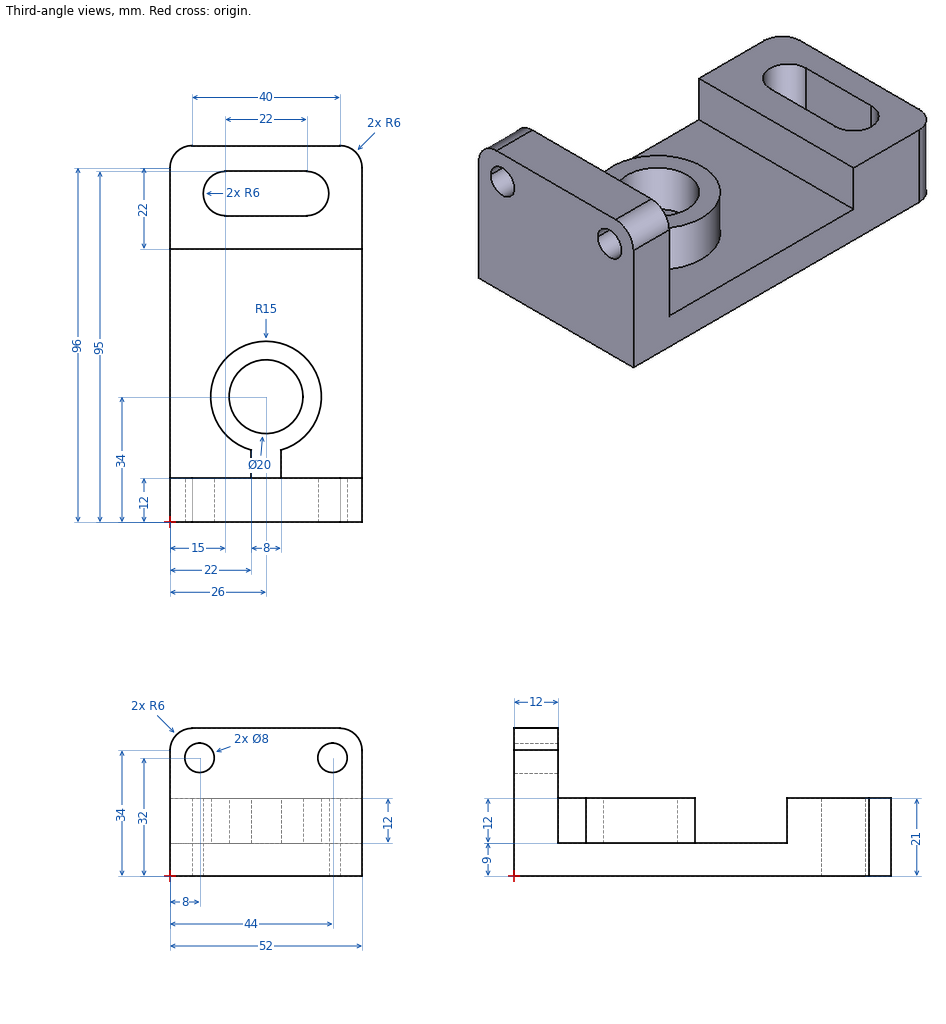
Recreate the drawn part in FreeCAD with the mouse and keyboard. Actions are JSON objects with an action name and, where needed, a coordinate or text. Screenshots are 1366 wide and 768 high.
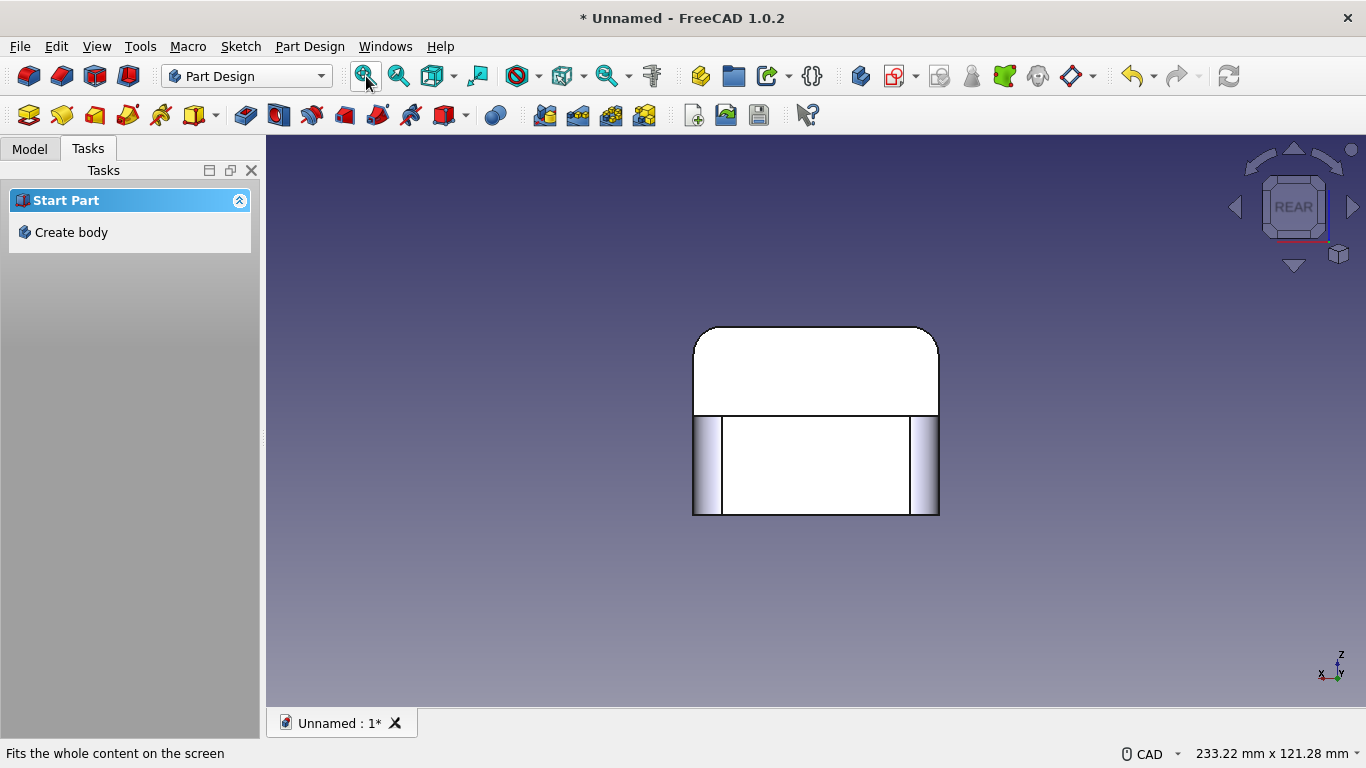
{"action": "left_click", "coordinate": [366, 76]}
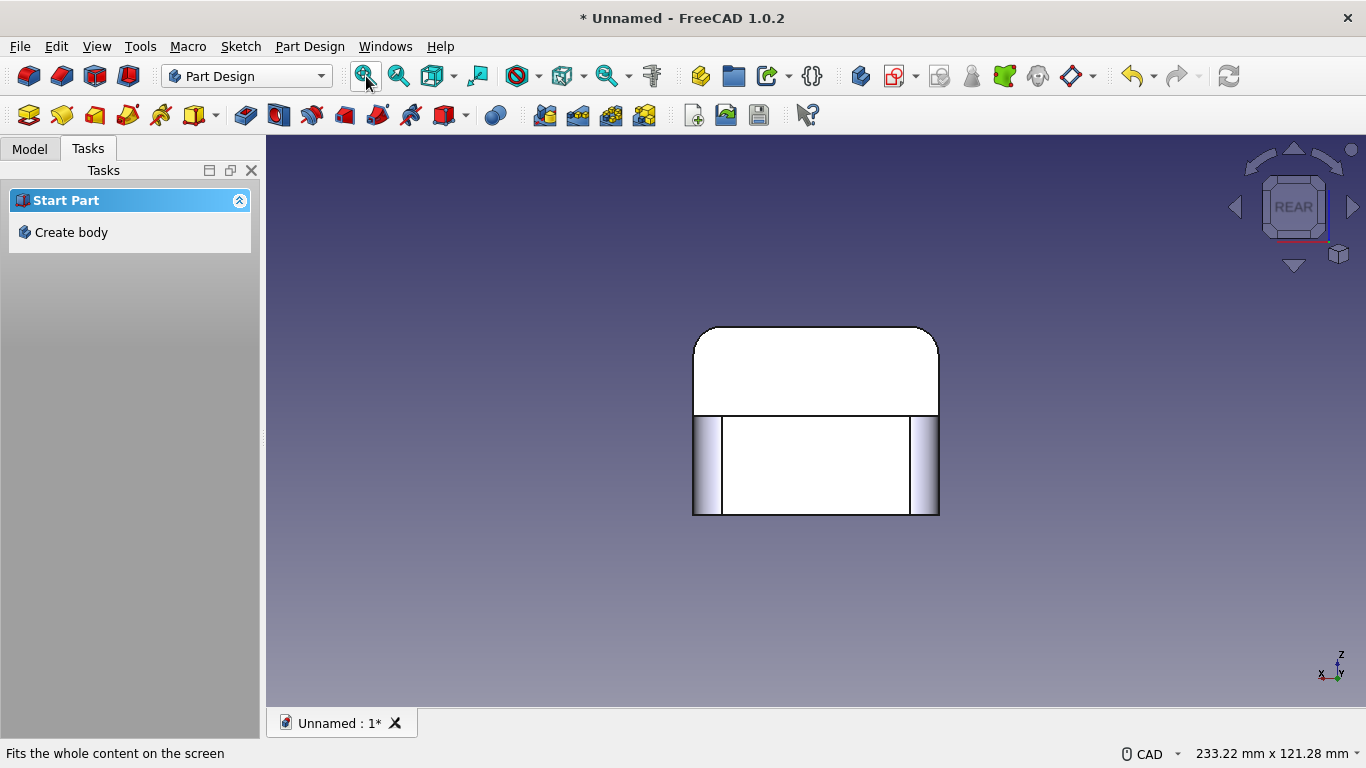
{"action": "left_click", "coordinate": [781, 399]}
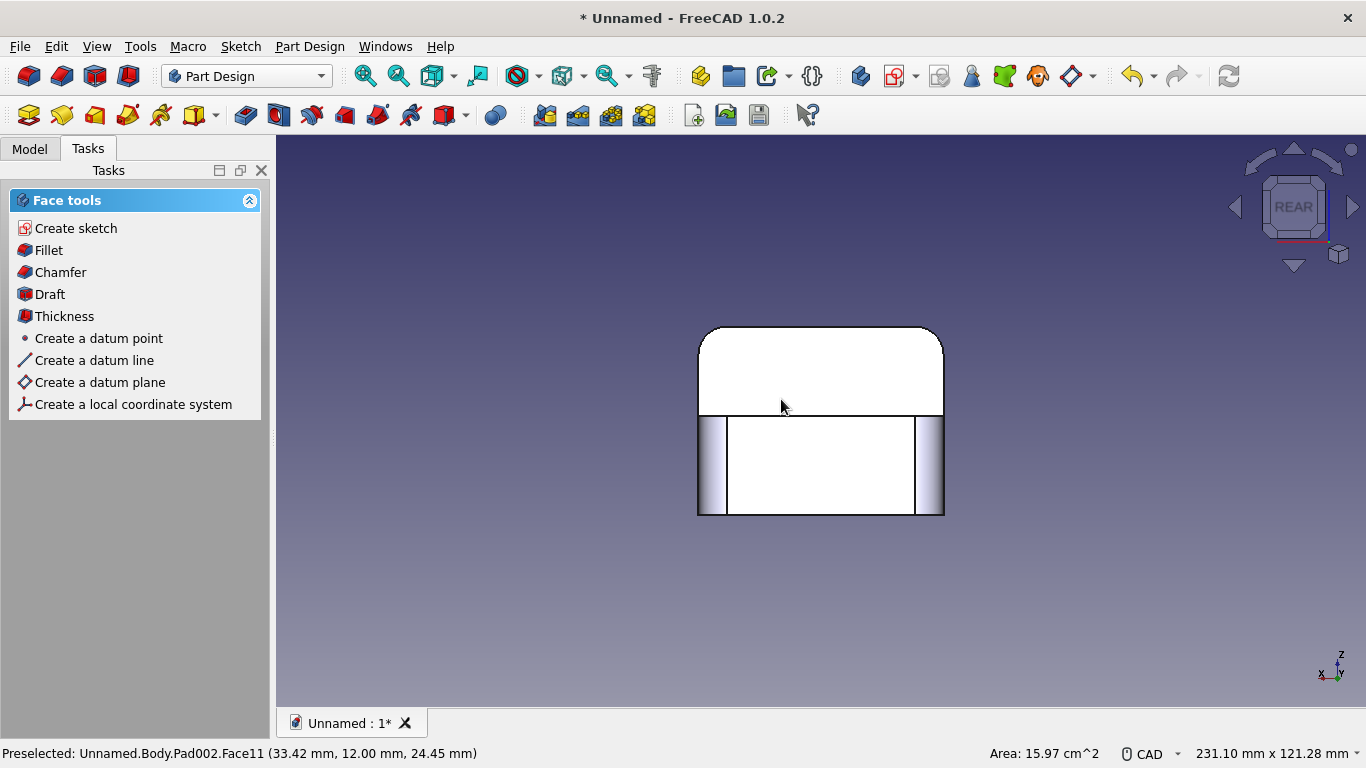
{"action": "left_click", "coordinate": [894, 76]}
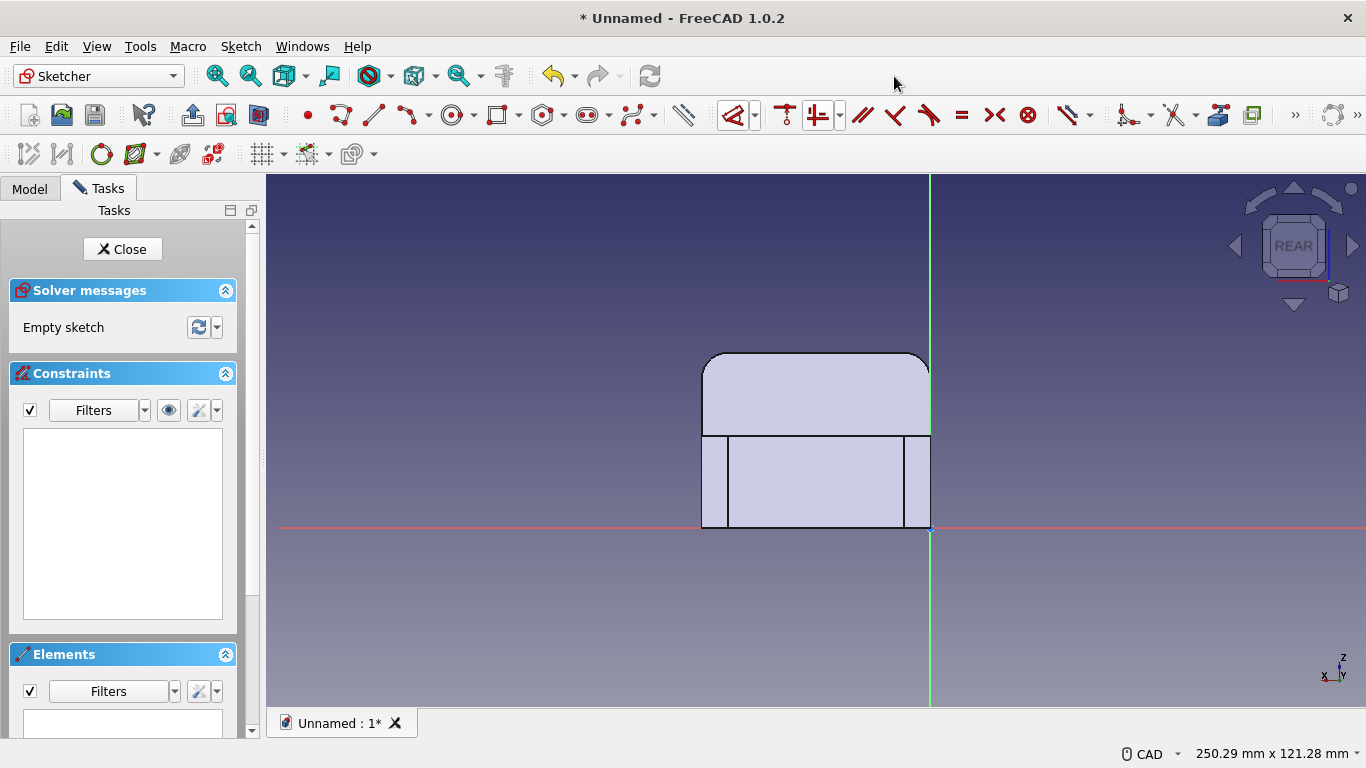
{"action": "scroll", "coordinate": [888, 456], "scroll_direction": "up", "scroll_amount": 4}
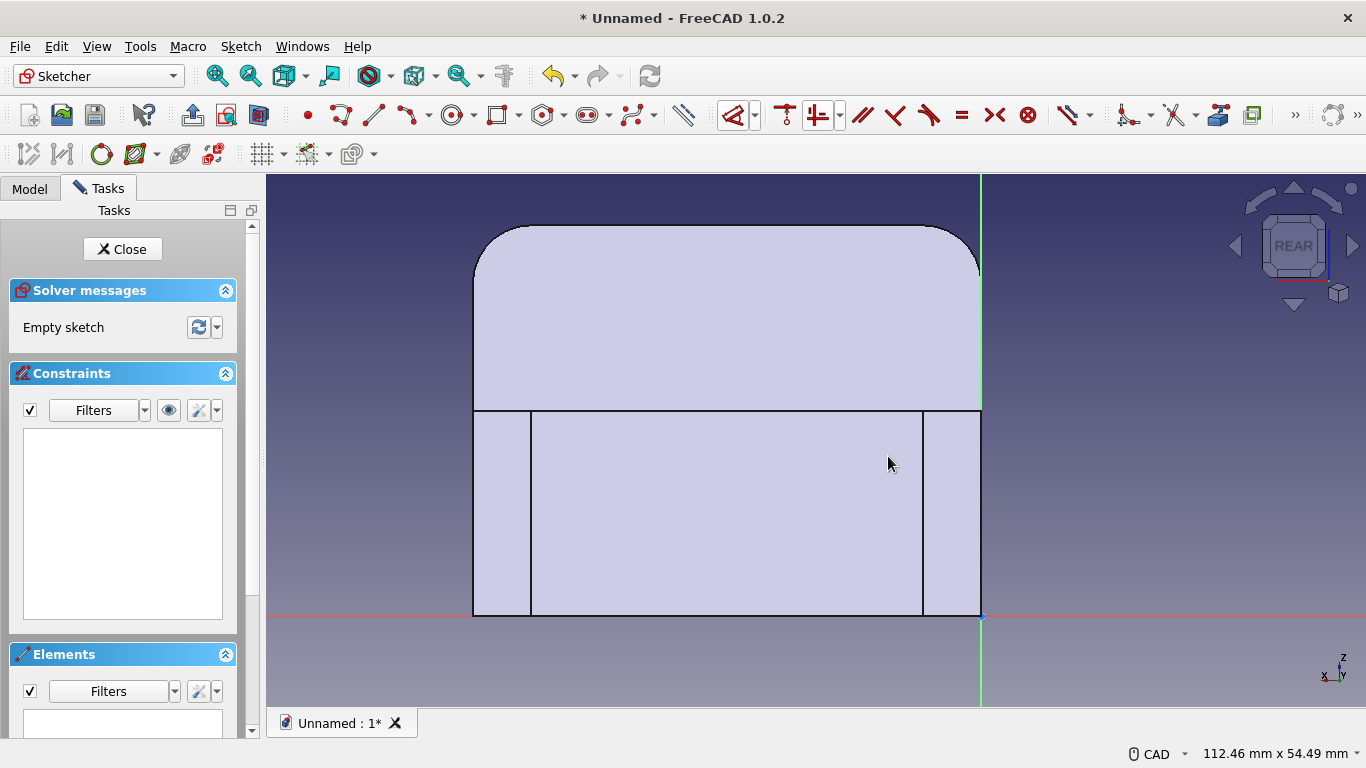
{"action": "left_click", "coordinate": [452, 116]}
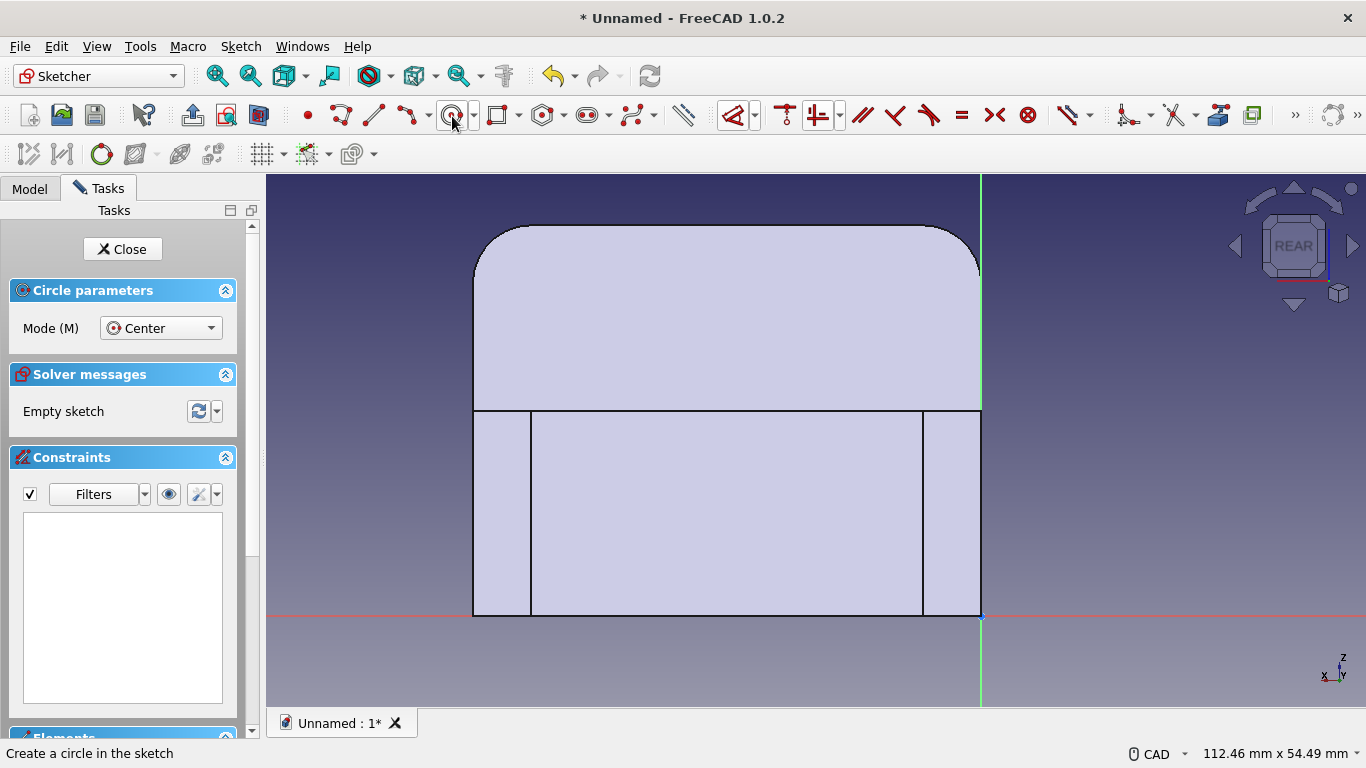
{"action": "left_click", "coordinate": [903, 303]}
{"action": "mouse_move", "coordinate": [931, 276]}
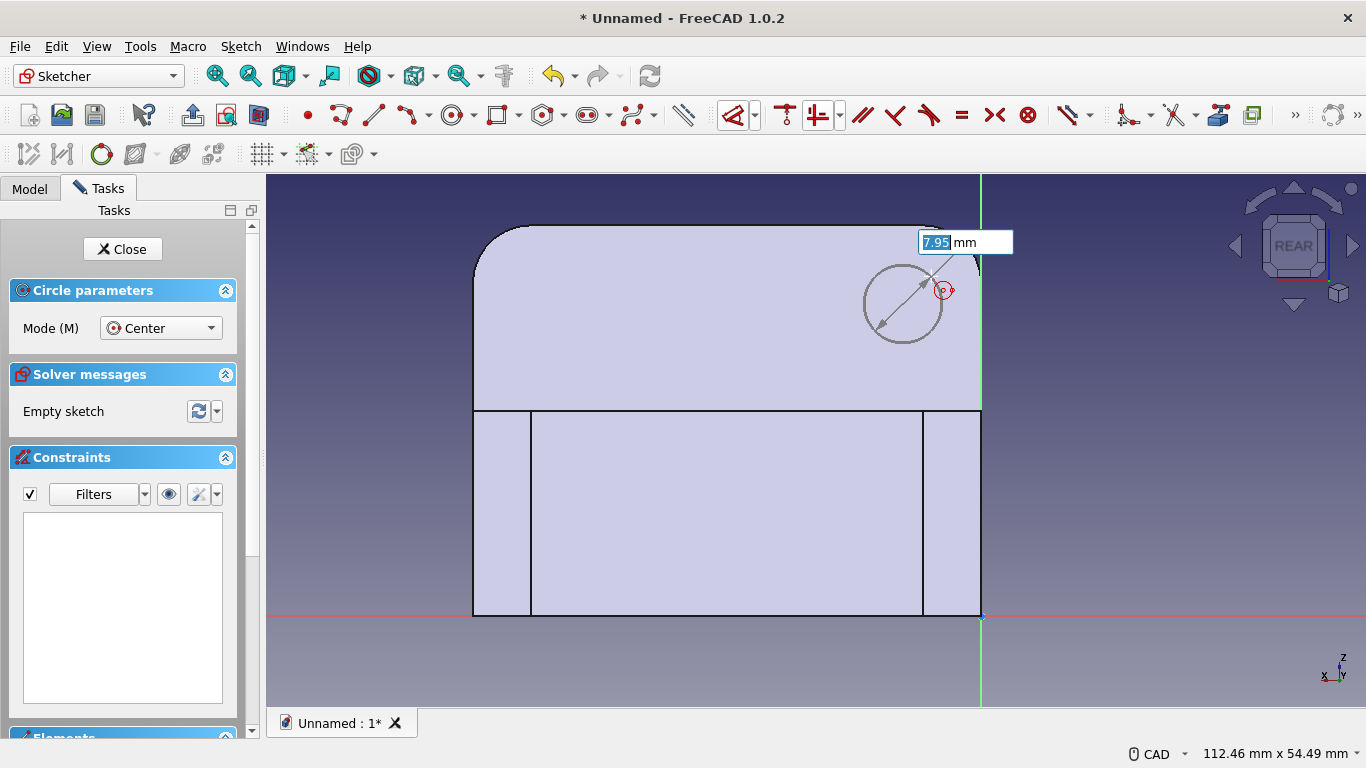
{"action": "type", "text": "8"}
{"action": "key", "text": "Return"}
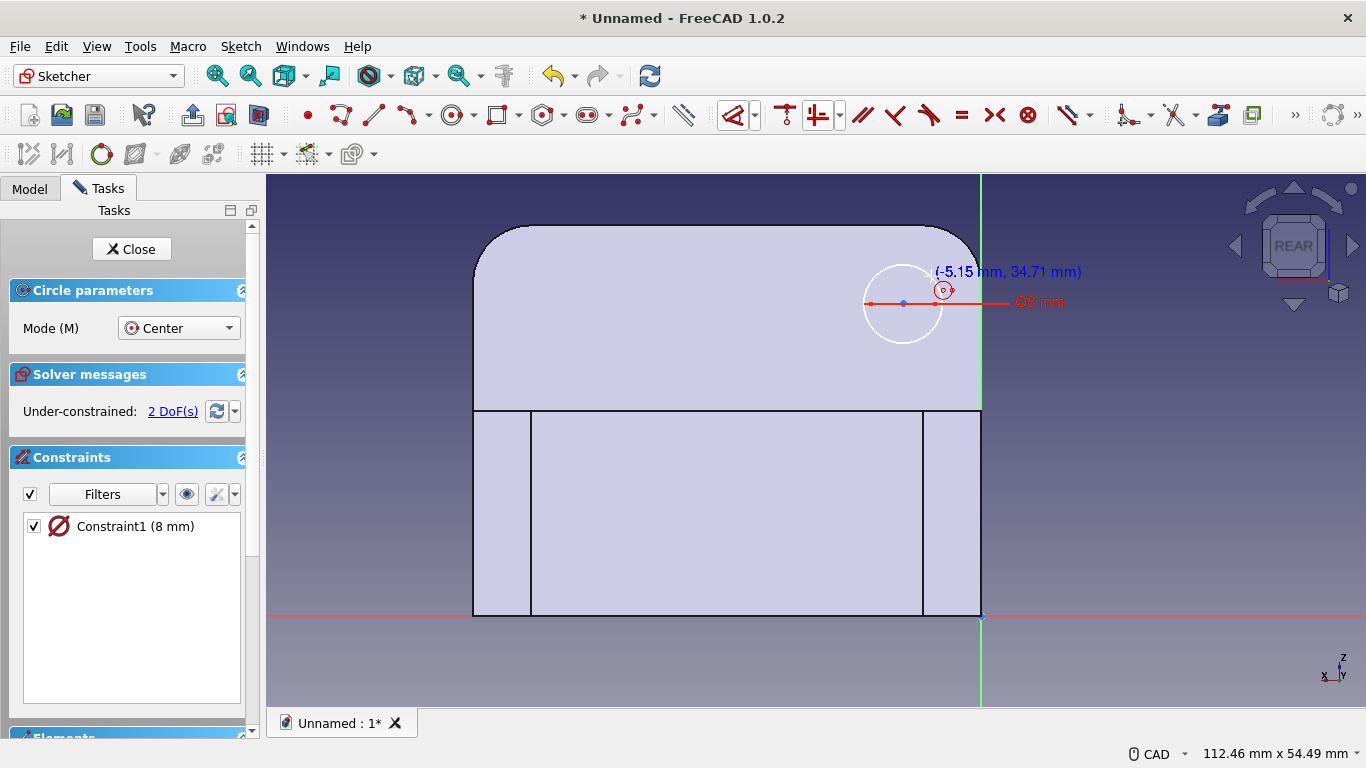
{"action": "left_click", "coordinate": [551, 303]}
{"action": "mouse_move", "coordinate": [579, 276]}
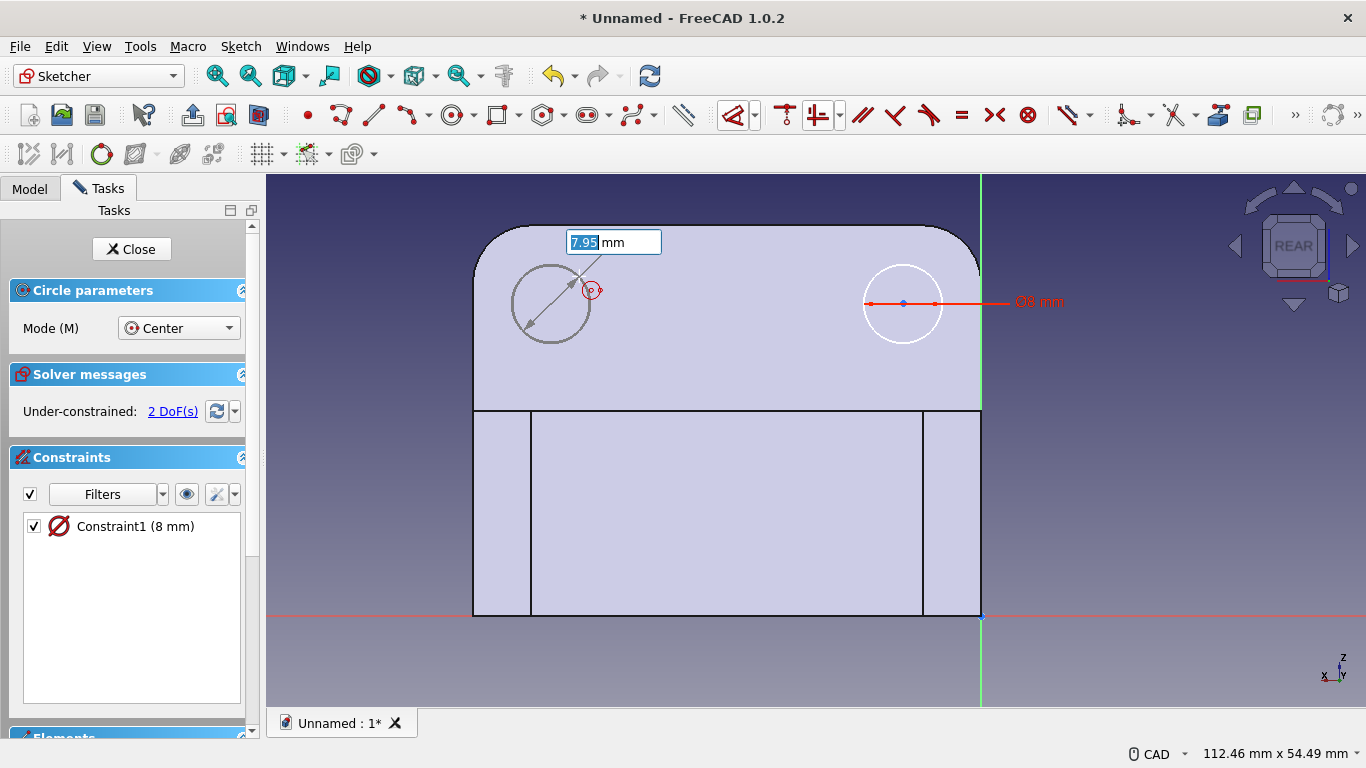
{"action": "type", "text": "8"}
{"action": "key", "text": "Return"}
{"action": "key", "text": "Escape"}